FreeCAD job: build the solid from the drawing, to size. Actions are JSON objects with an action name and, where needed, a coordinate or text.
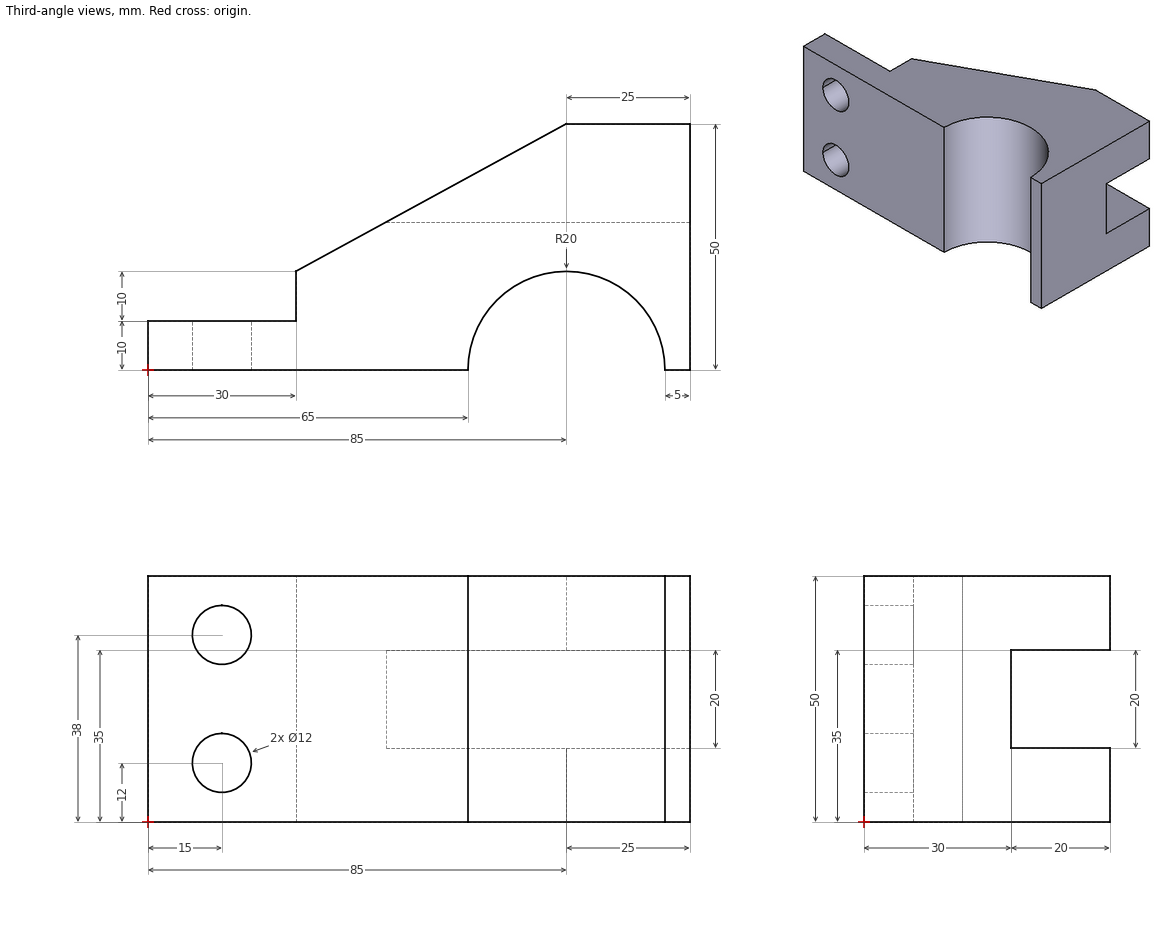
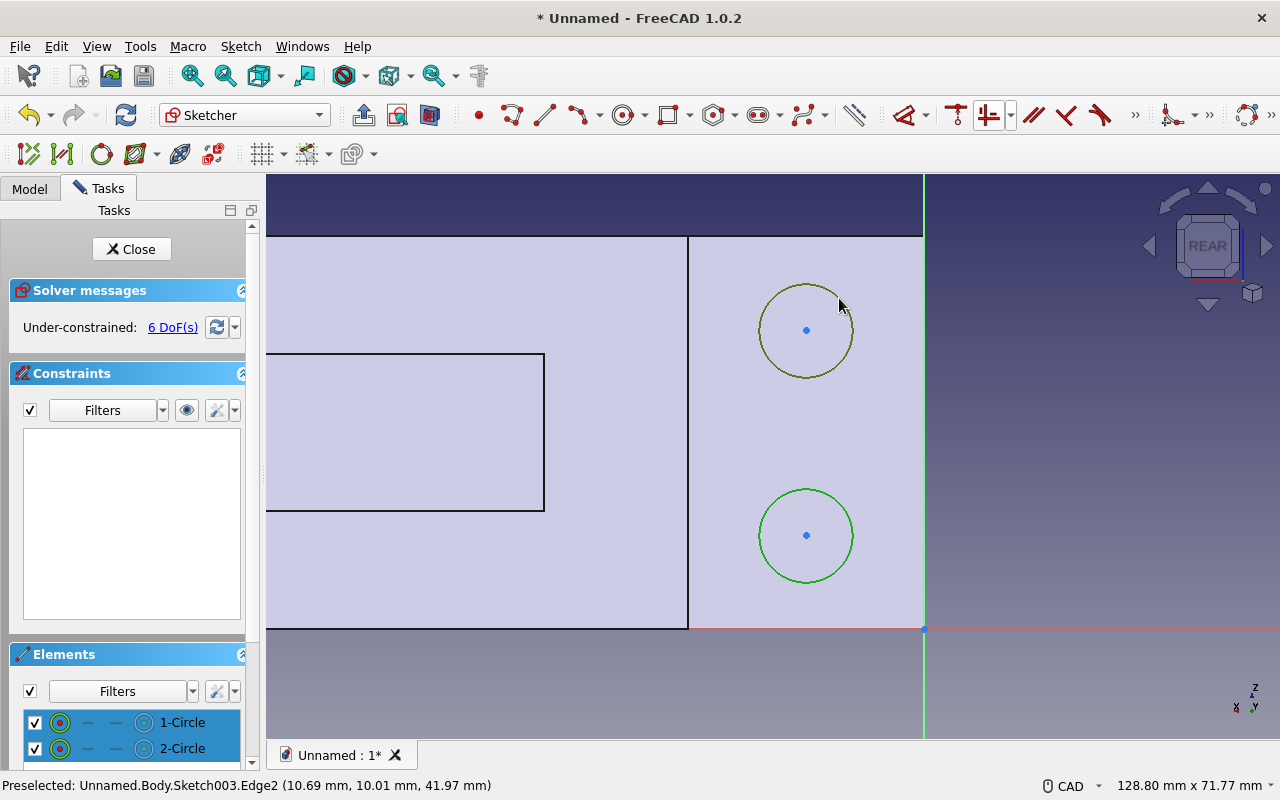
{"action": "key", "text": "e"}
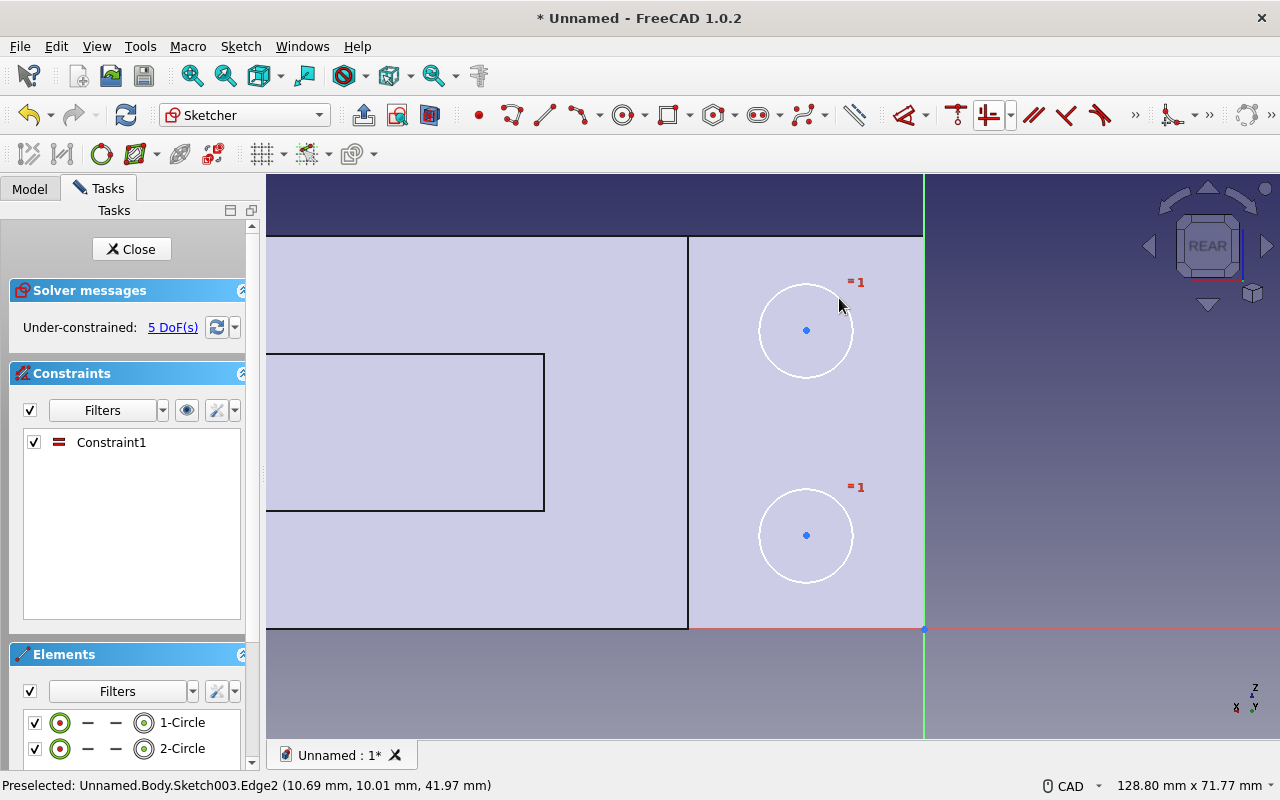
{"action": "left_click", "coordinate": [806, 536]}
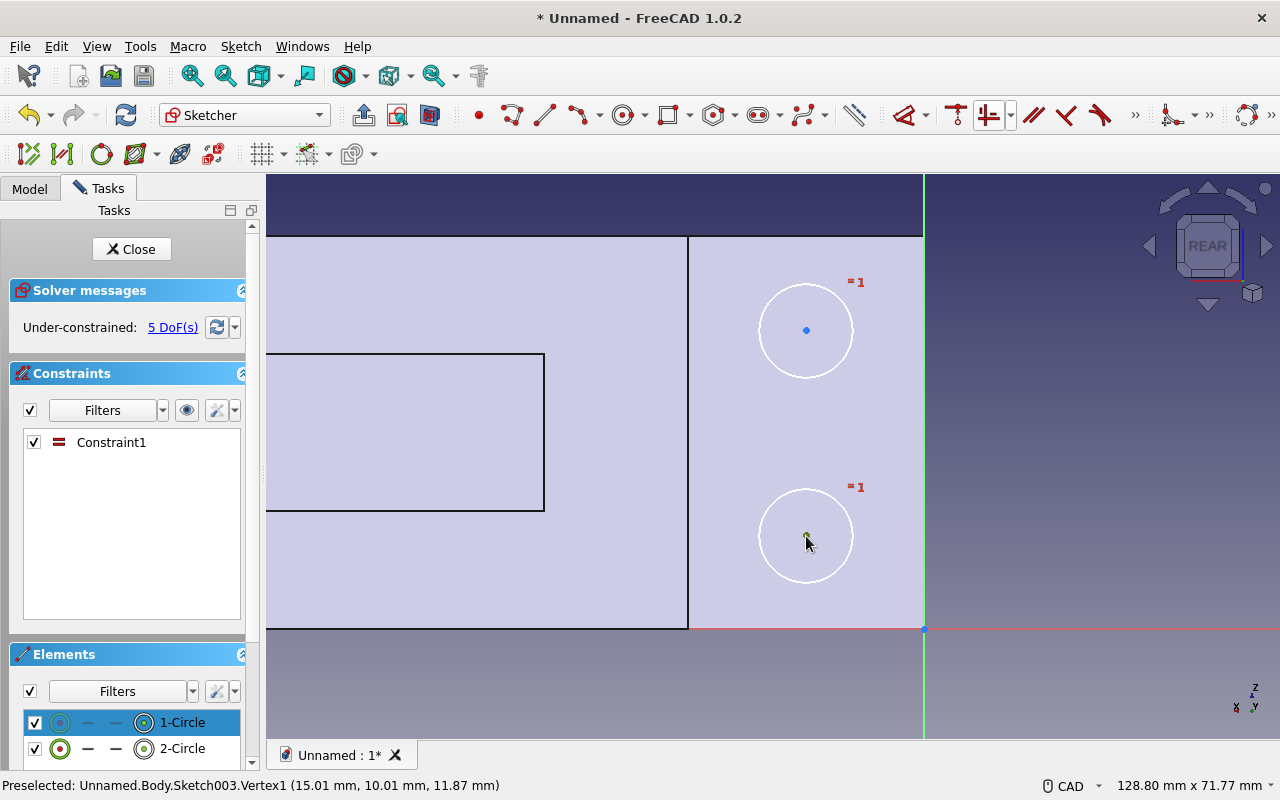
{"action": "left_click", "coordinate": [806, 331]}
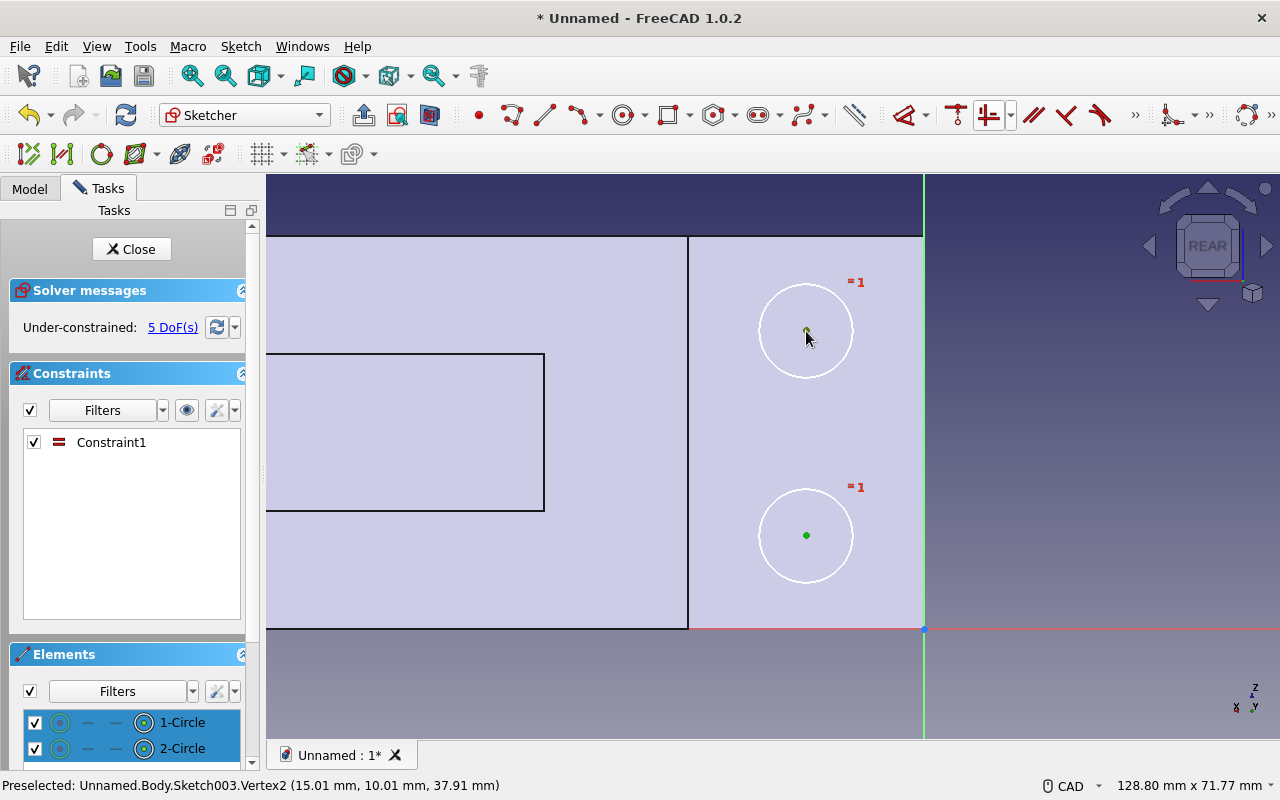
{"action": "key", "text": "v"}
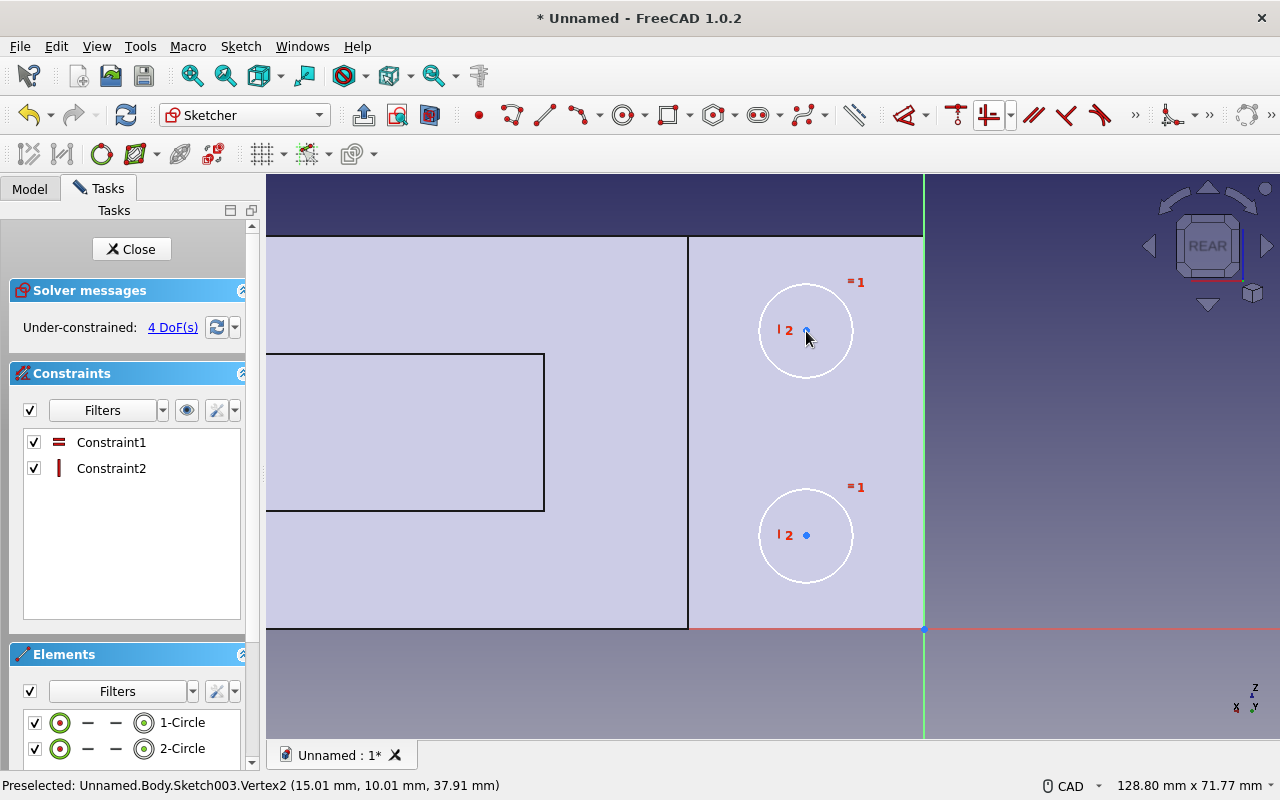
{"action": "left_click", "coordinate": [904, 116]}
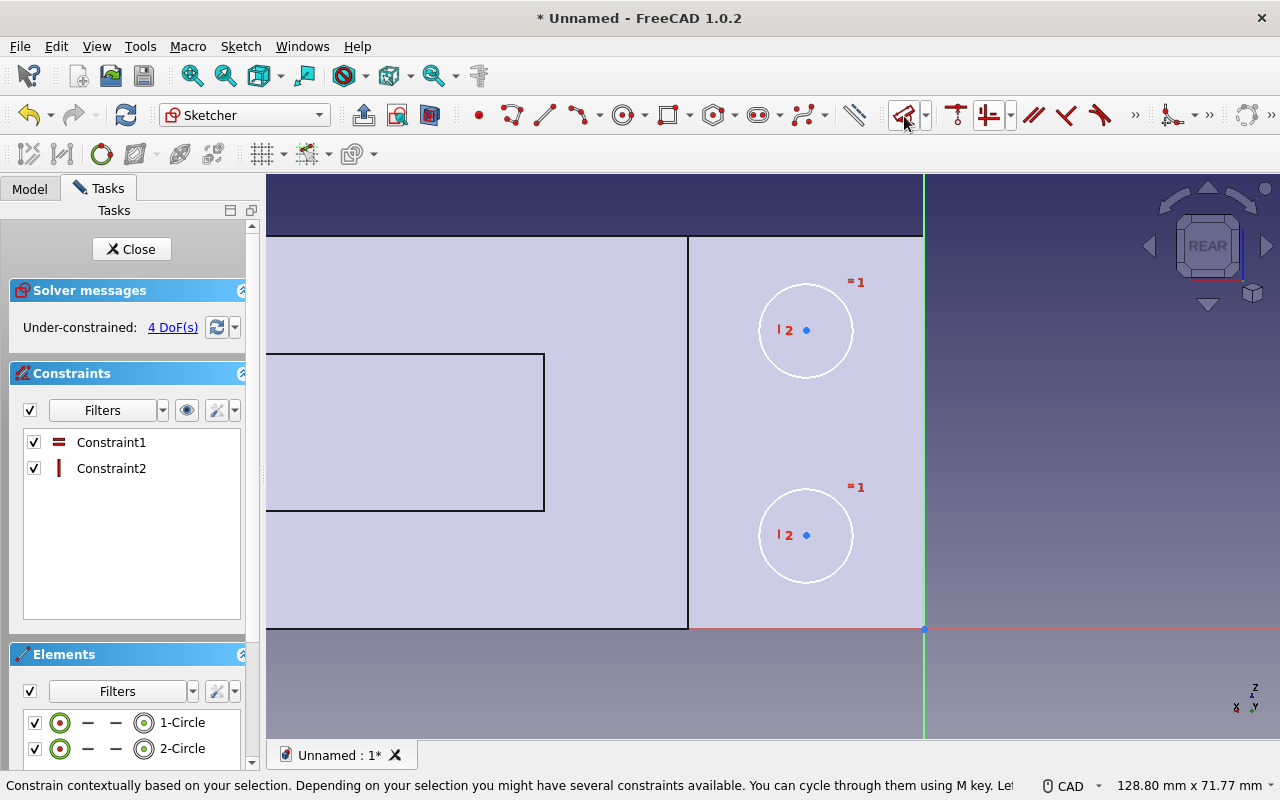
{"action": "left_click", "coordinate": [839, 503]}
{"action": "left_click", "coordinate": [862, 480]}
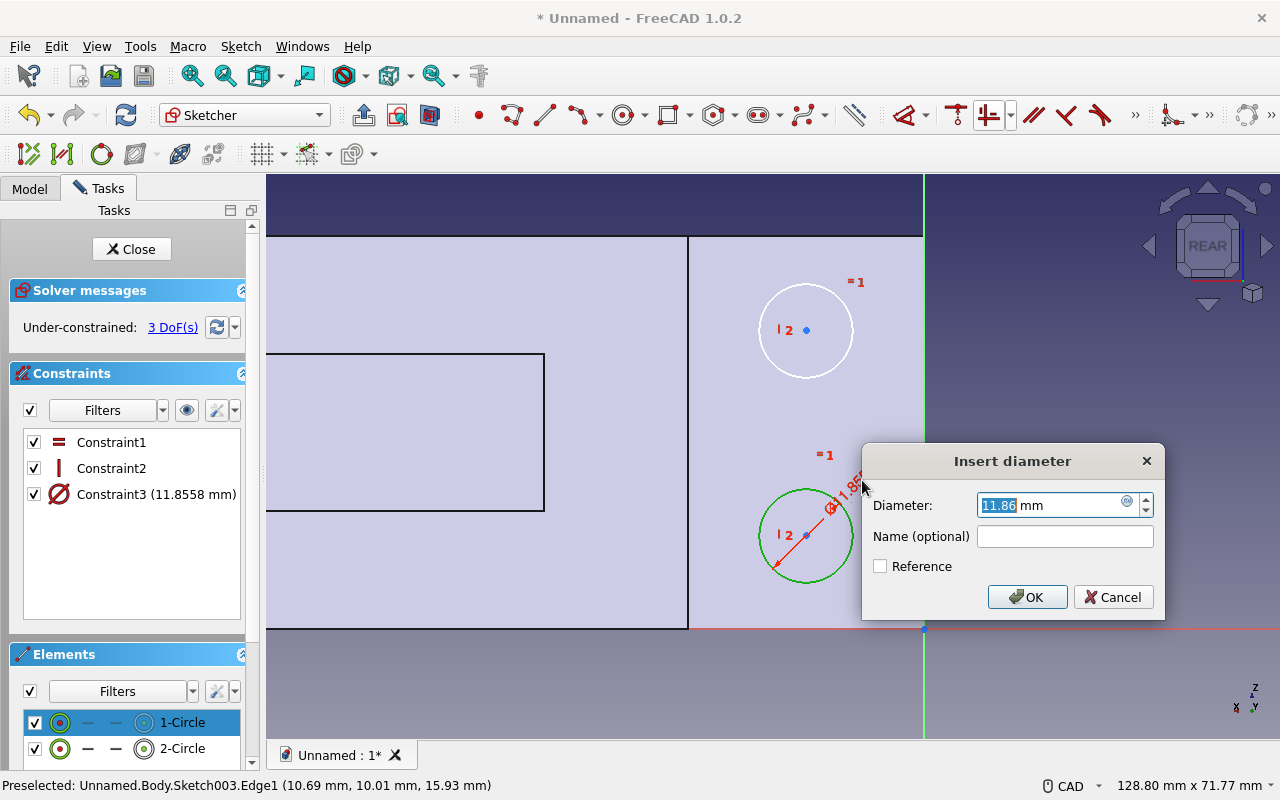
{"action": "type", "text": "12"}
{"action": "key", "text": "Return"}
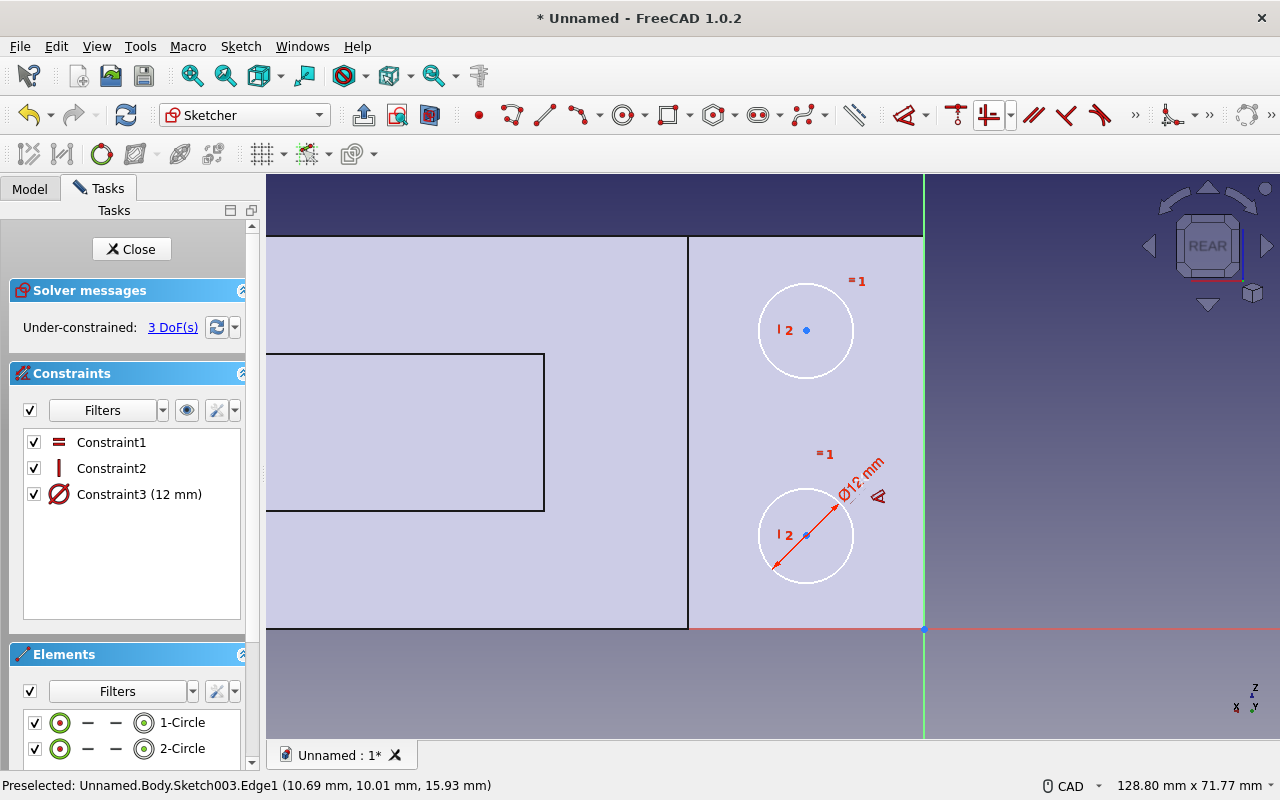
{"action": "left_click", "coordinate": [806, 536]}
{"action": "left_click", "coordinate": [865, 663]}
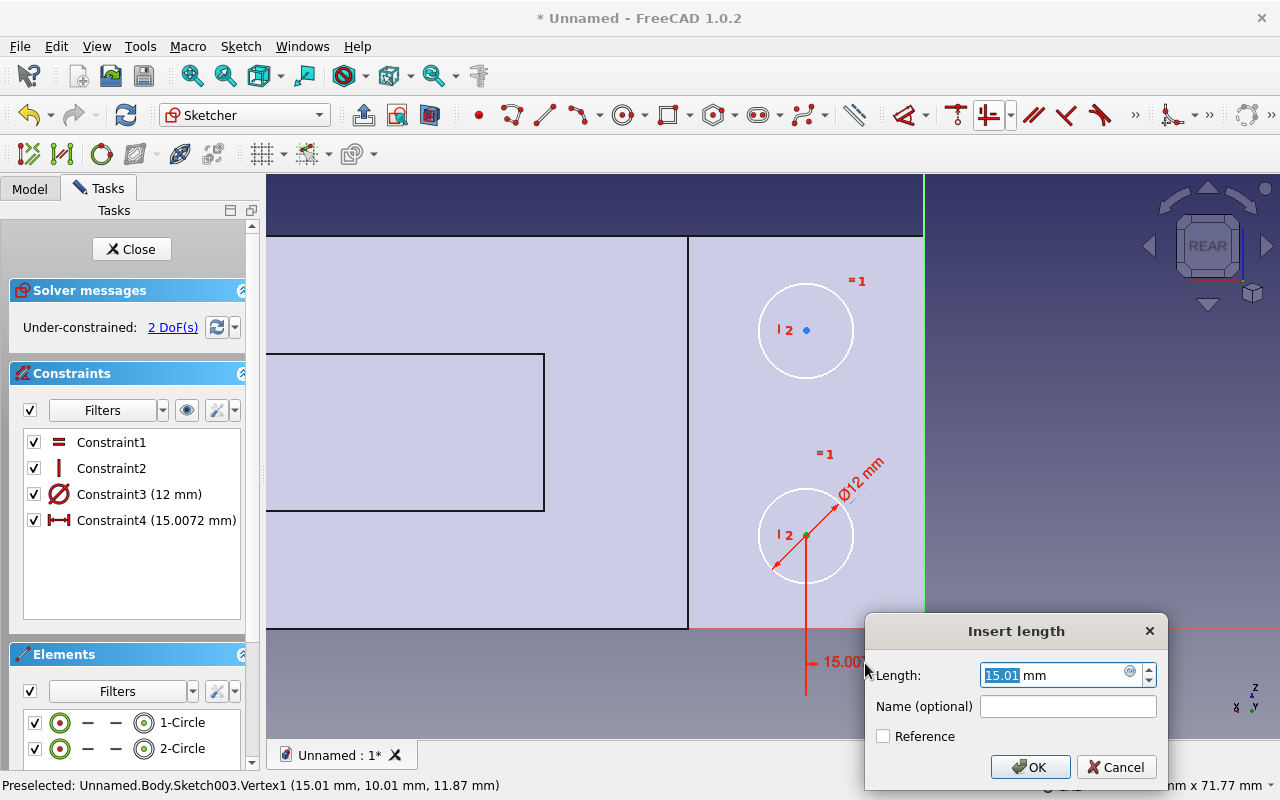
{"action": "type", "text": "15"}
{"action": "key", "text": "Return"}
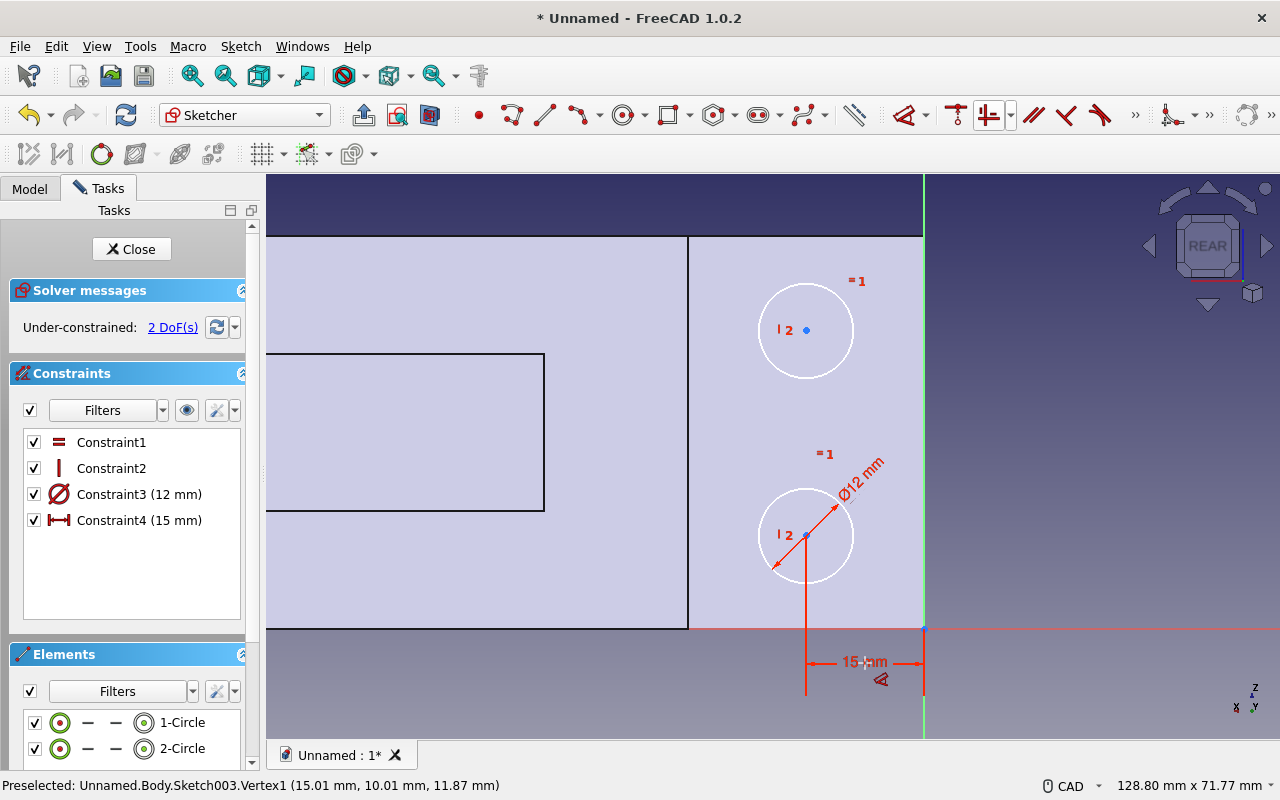
{"action": "left_click", "coordinate": [806, 536]}
{"action": "left_click", "coordinate": [958, 583]}